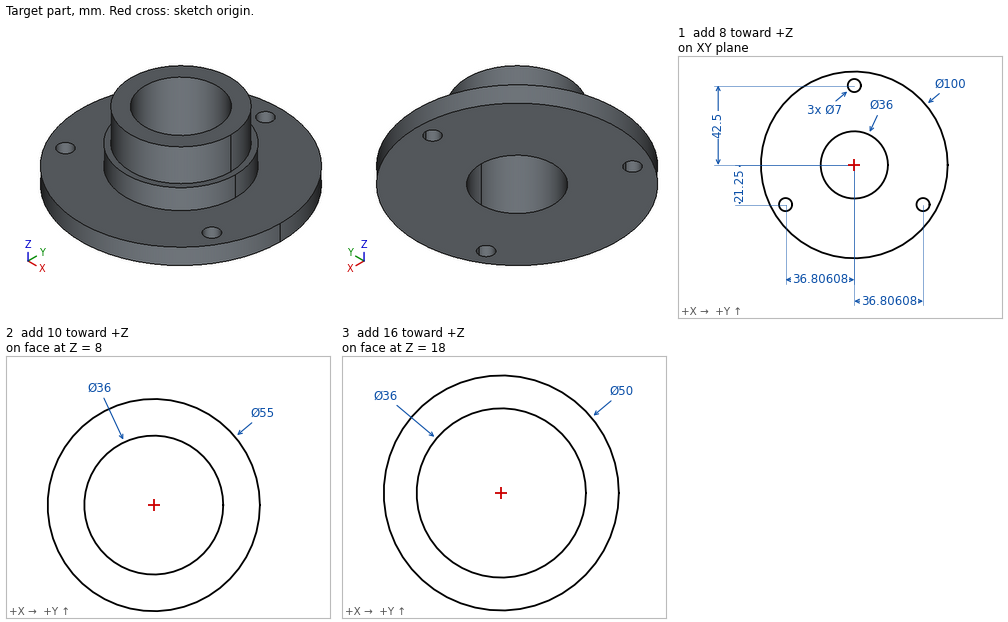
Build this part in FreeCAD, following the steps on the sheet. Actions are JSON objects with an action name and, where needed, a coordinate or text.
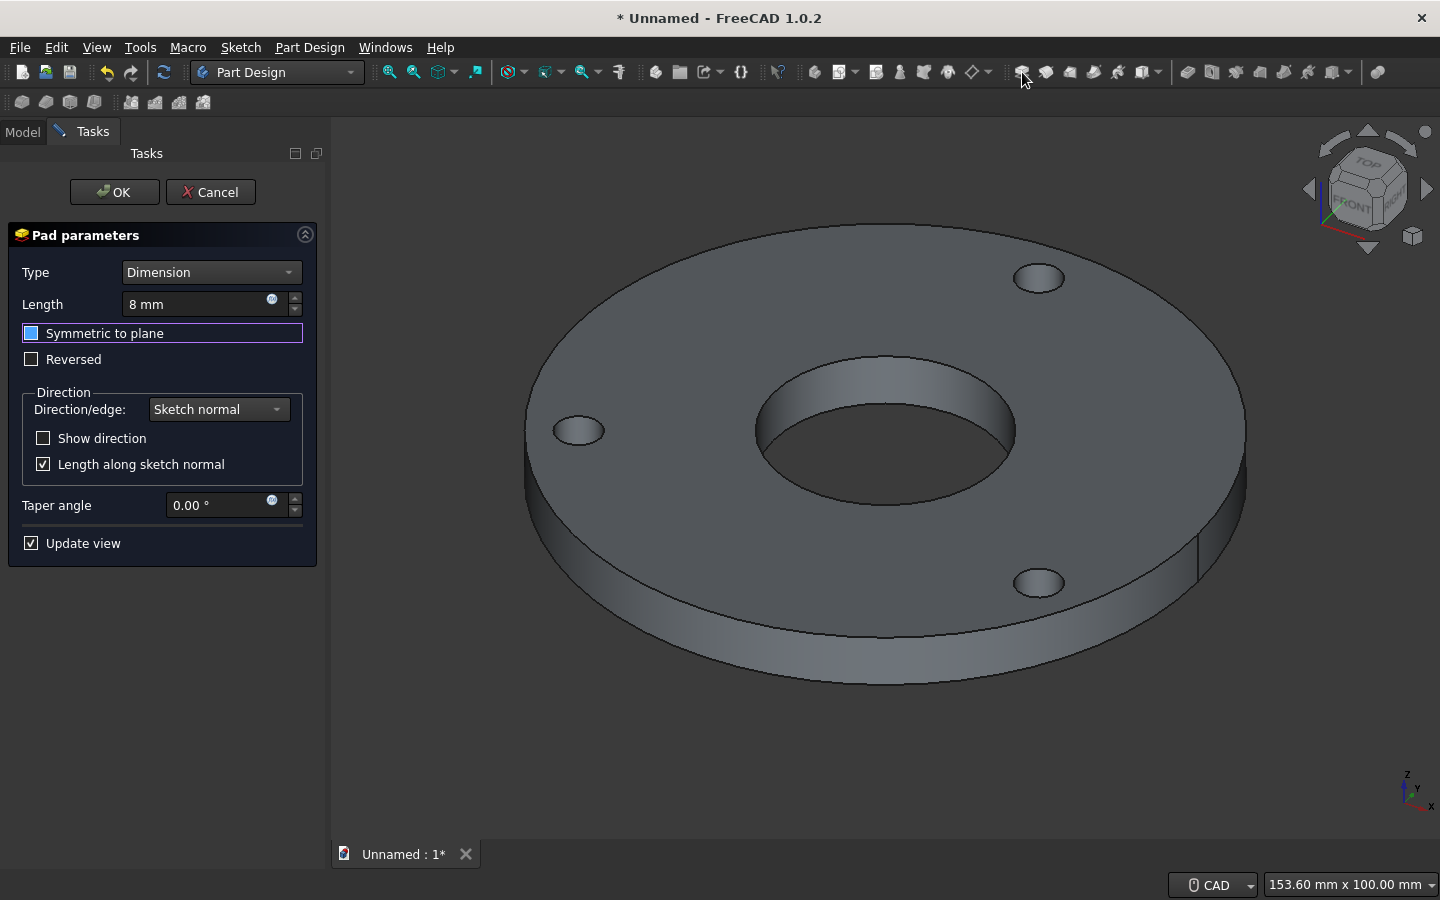
{"action": "left_click", "coordinate": [115, 192]}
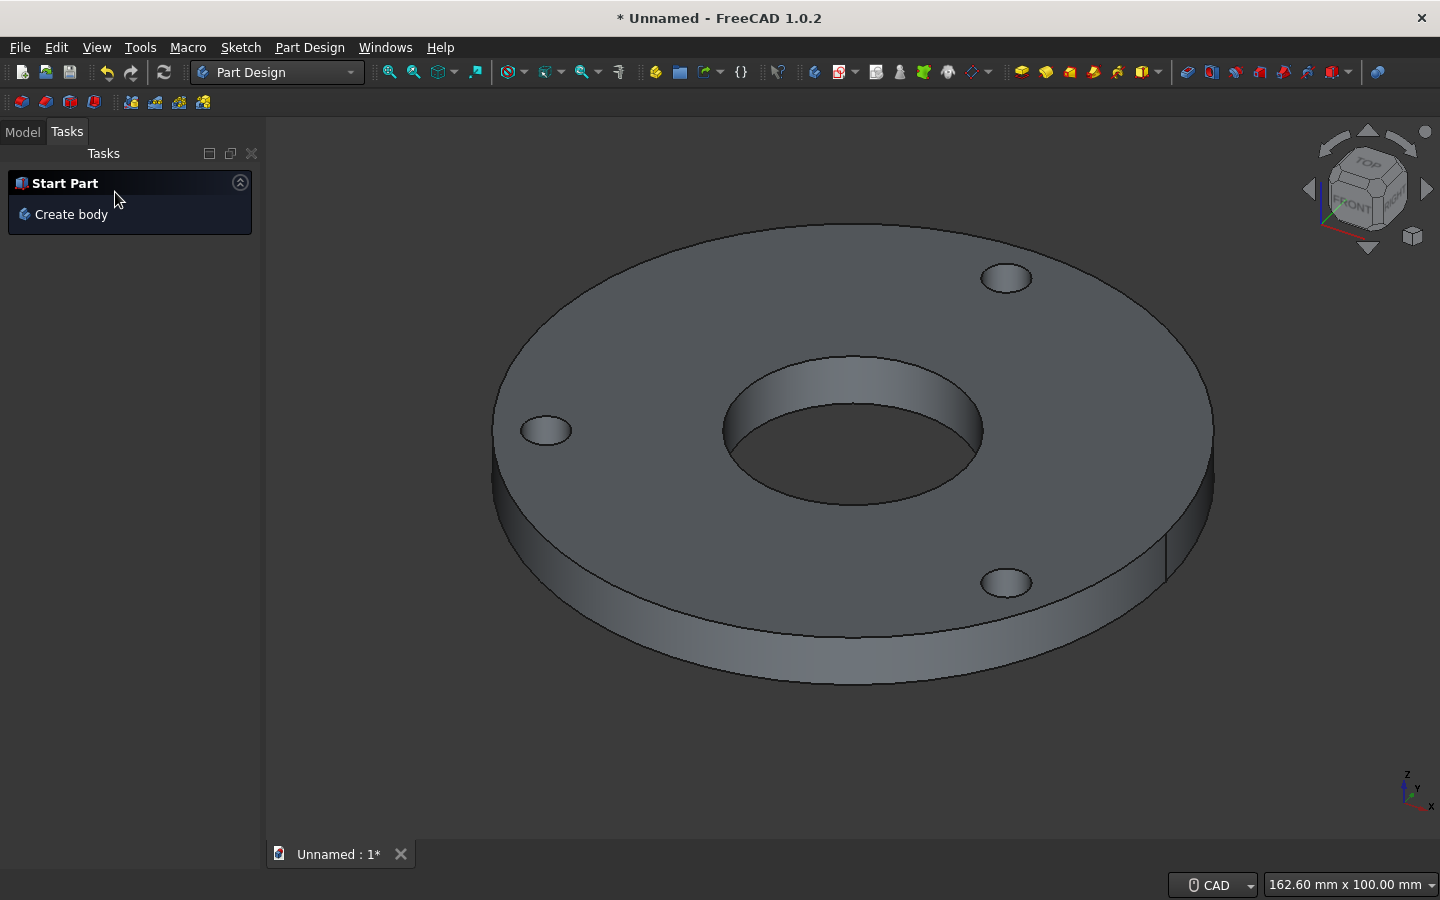
{"action": "left_click", "coordinate": [726, 319]}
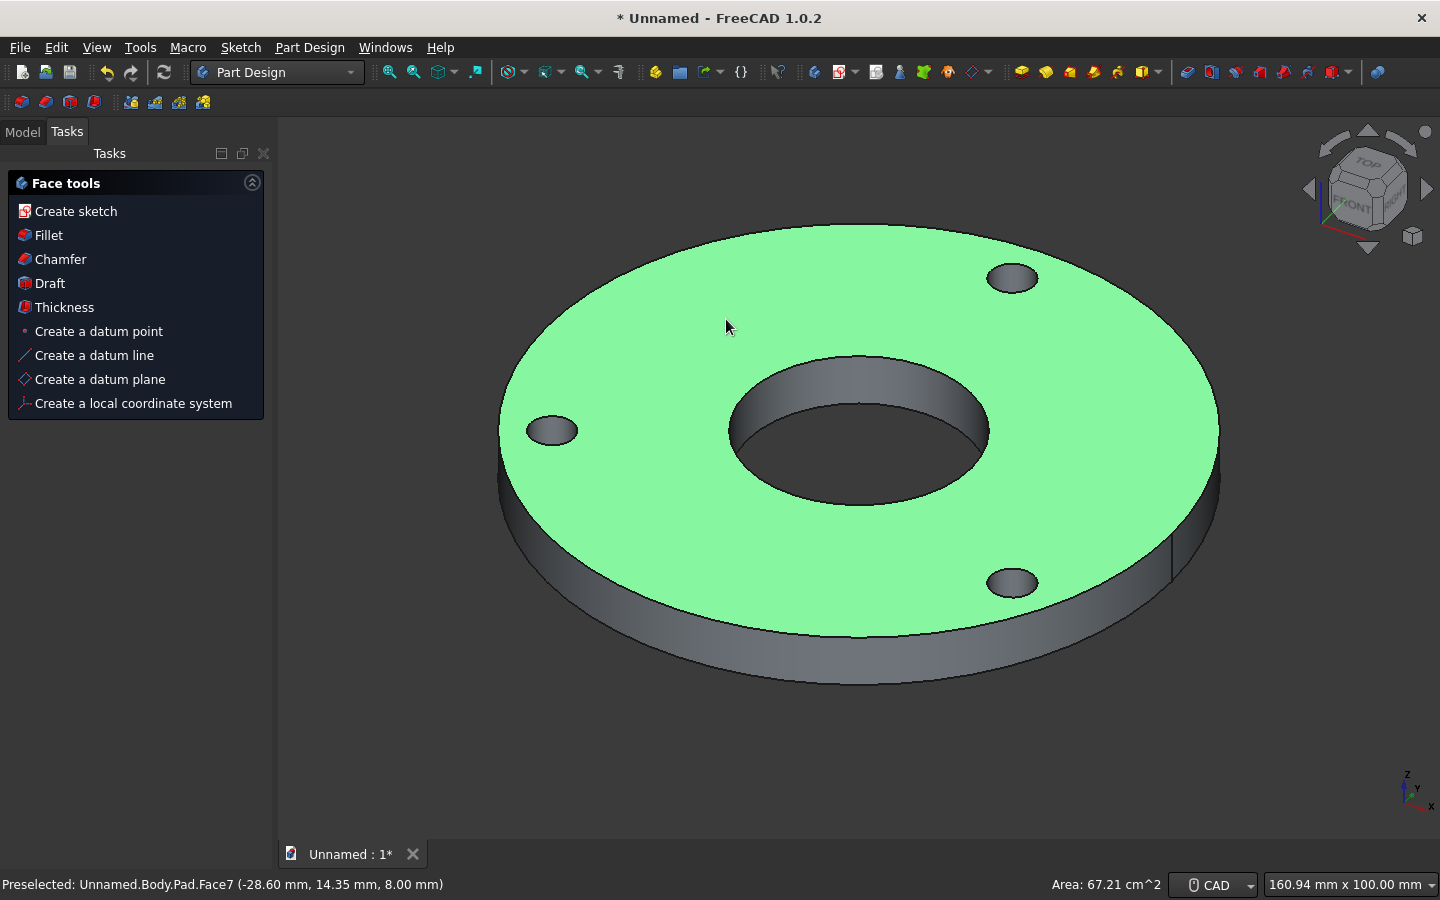
{"action": "left_click", "coordinate": [840, 72]}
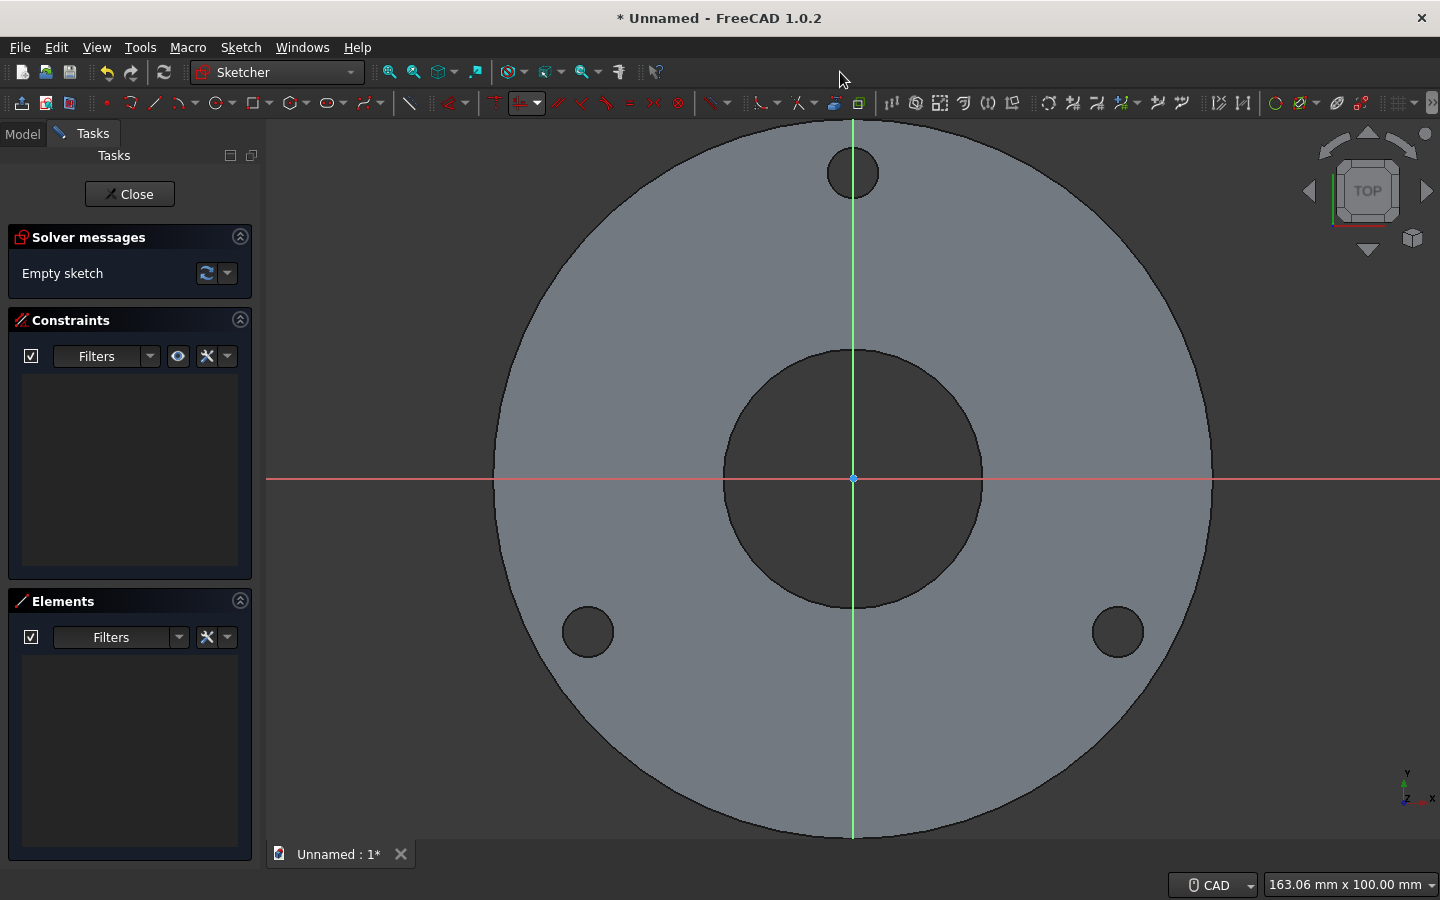
{"action": "left_click", "coordinate": [216, 104]}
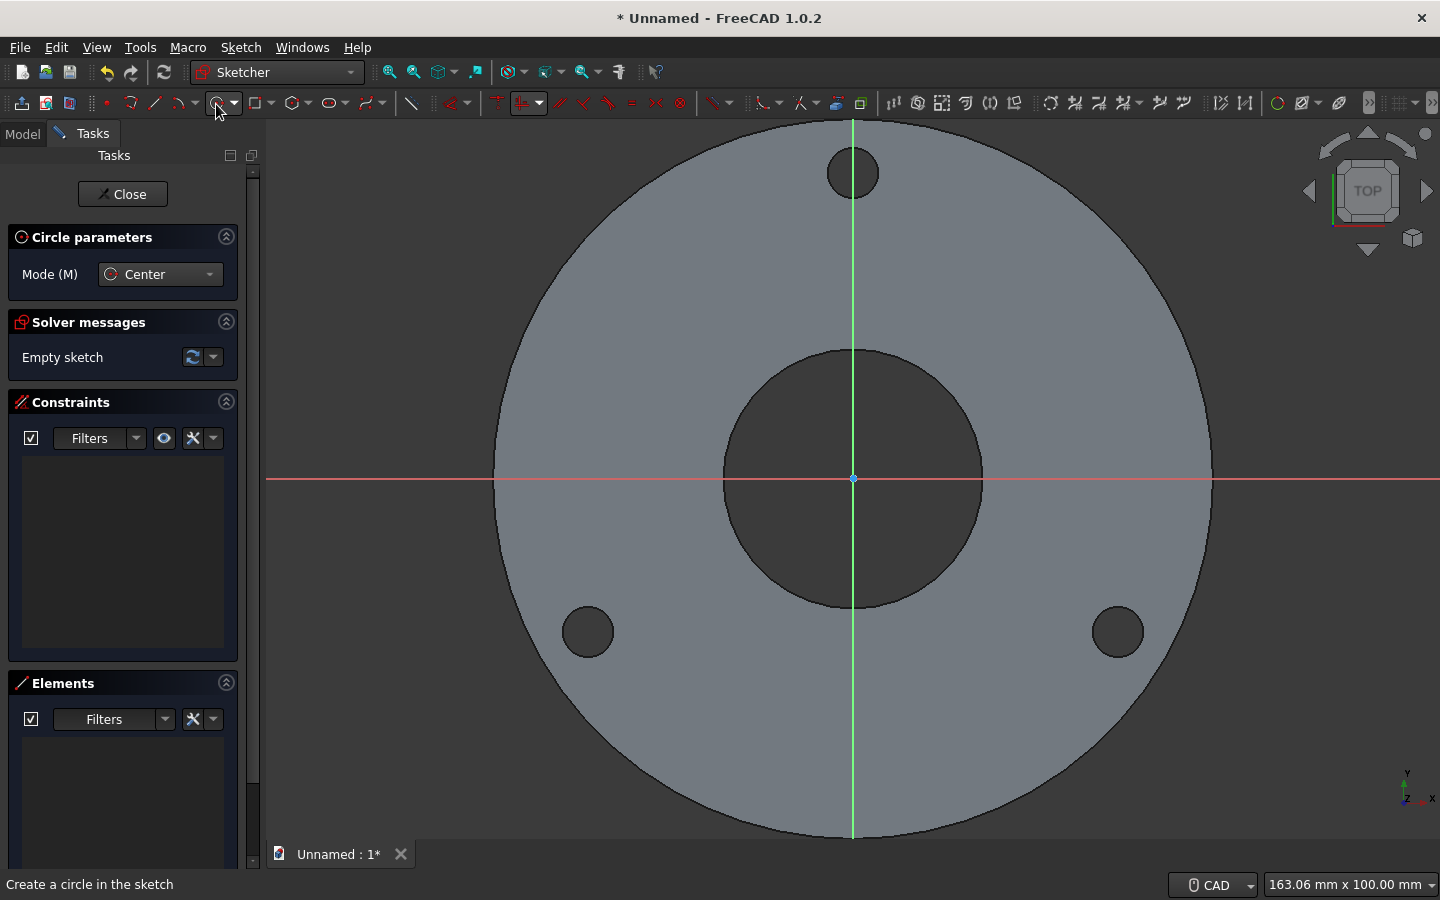
{"action": "left_click", "coordinate": [853, 479]}
{"action": "left_click", "coordinate": [993, 339]}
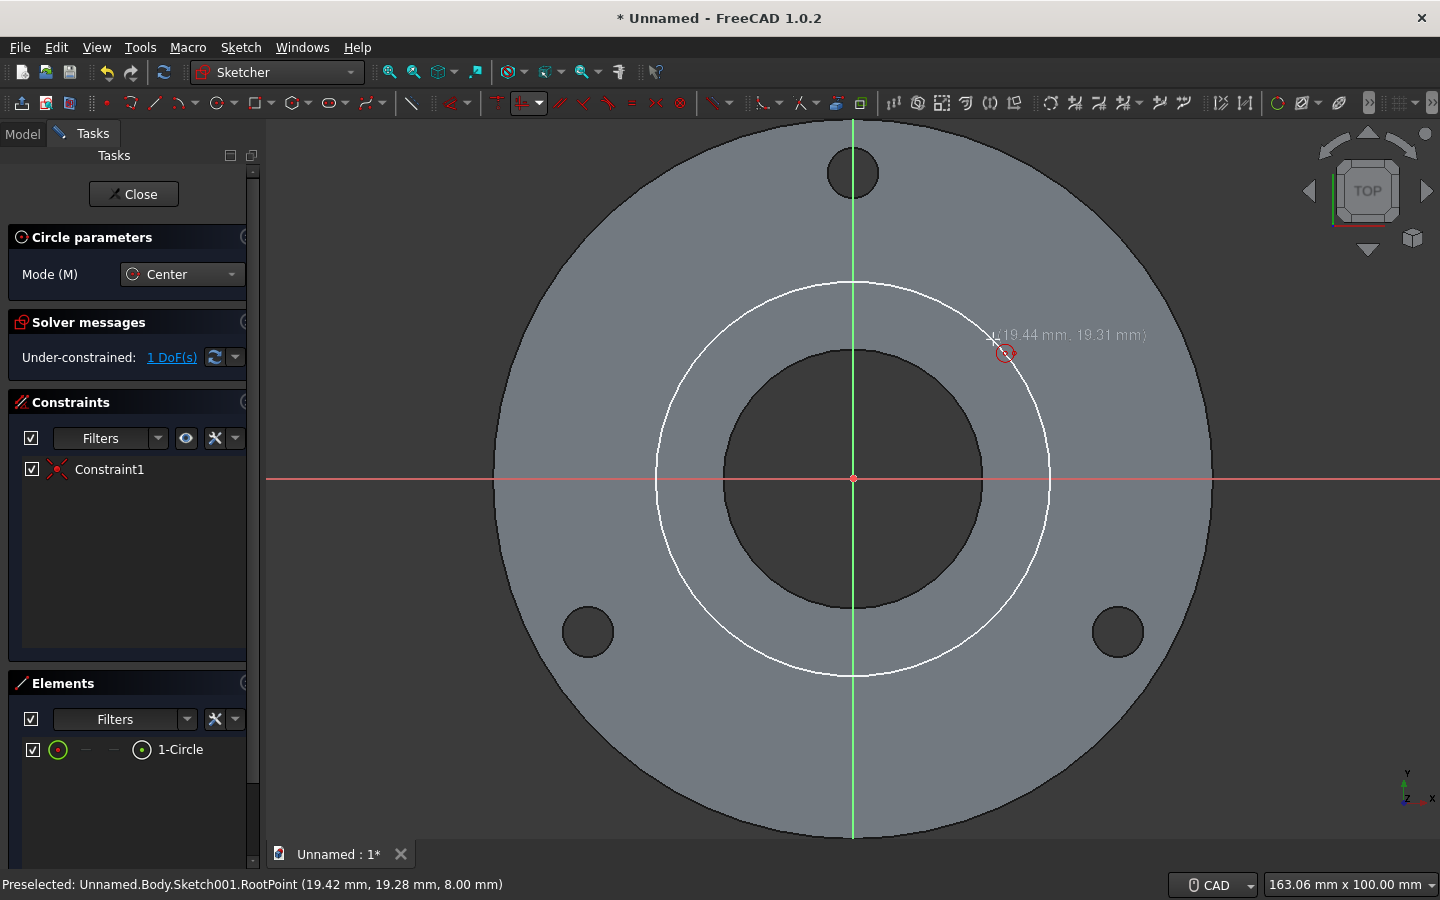
{"action": "left_click", "coordinate": [853, 479]}
{"action": "left_click", "coordinate": [945, 387]}
{"action": "key", "text": "Escape"}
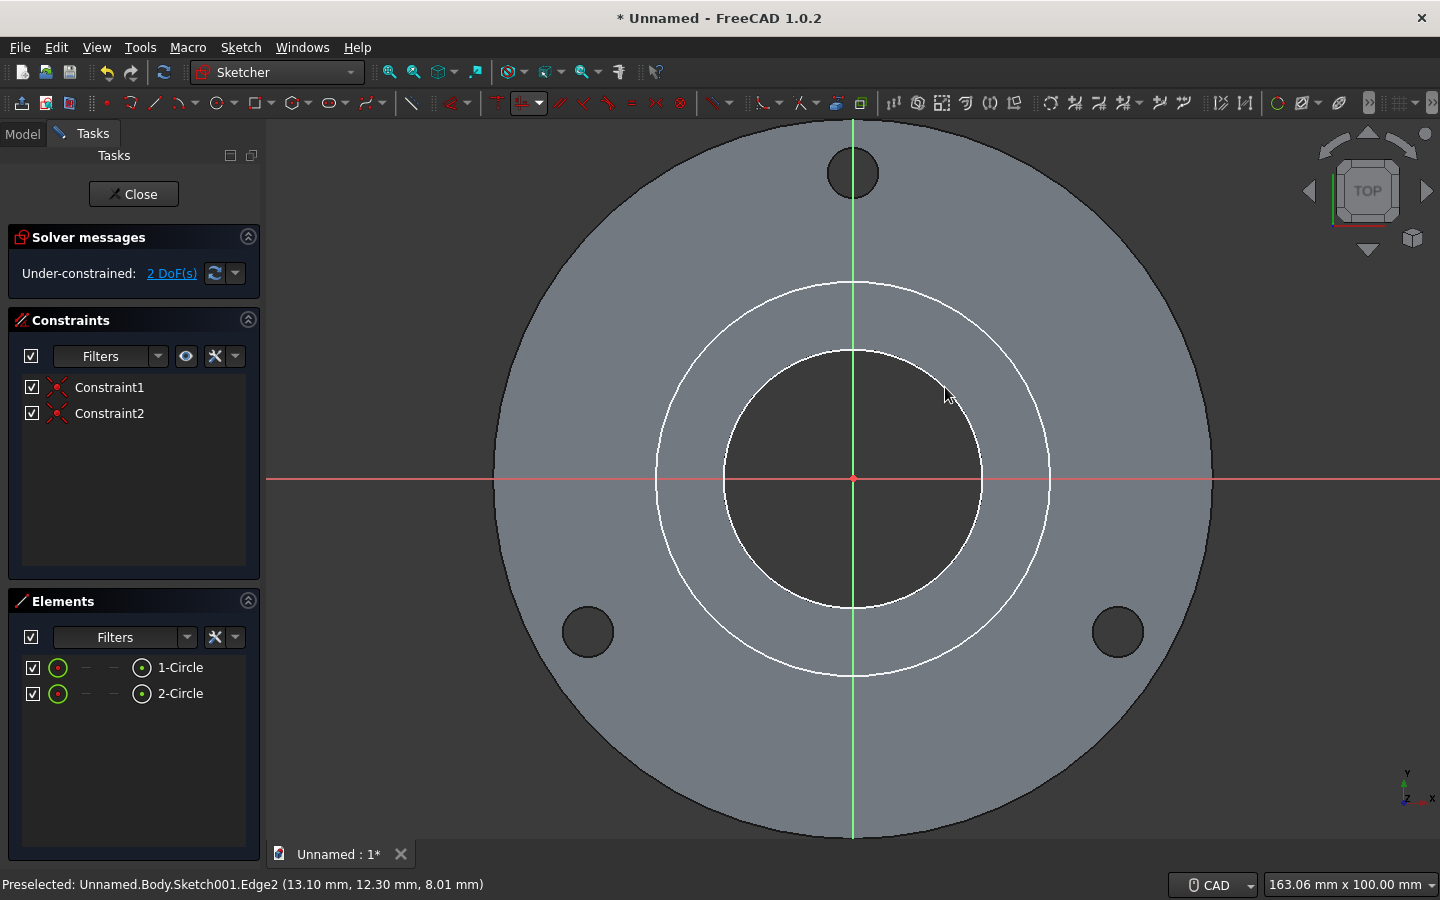
{"action": "left_click", "coordinate": [450, 104]}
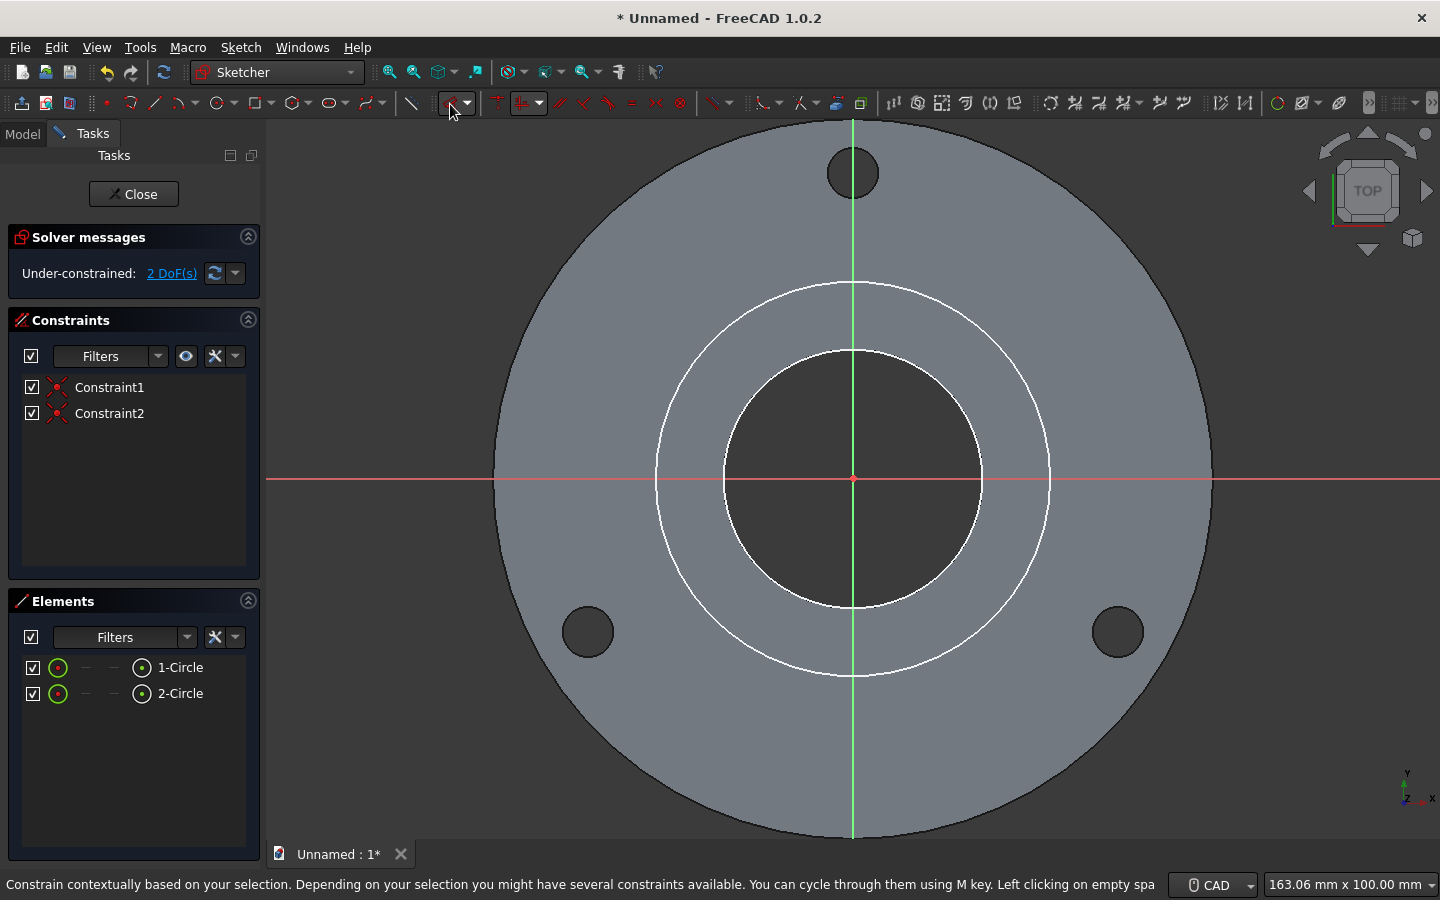
{"action": "left_click", "coordinate": [992, 339]}
{"action": "left_click", "coordinate": [1015, 316]}